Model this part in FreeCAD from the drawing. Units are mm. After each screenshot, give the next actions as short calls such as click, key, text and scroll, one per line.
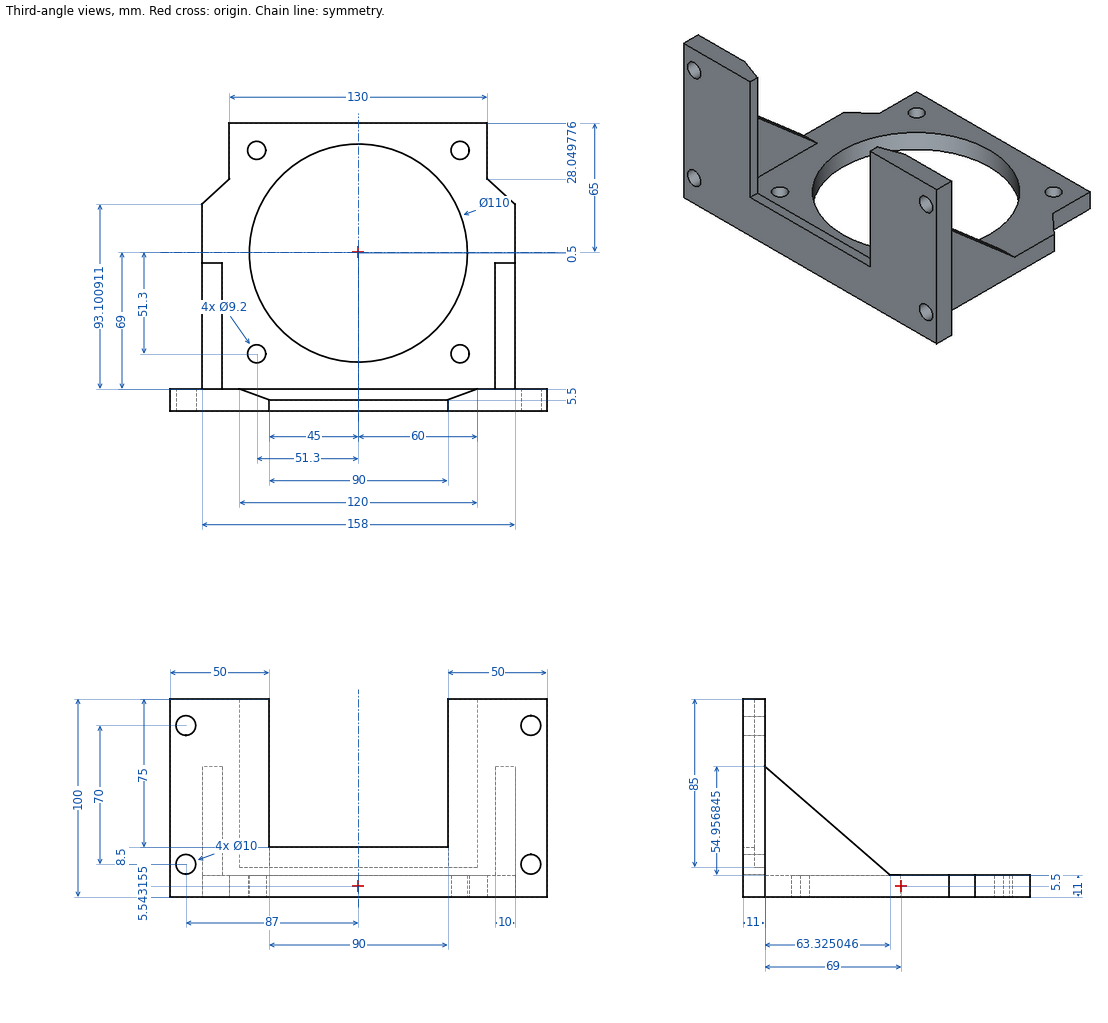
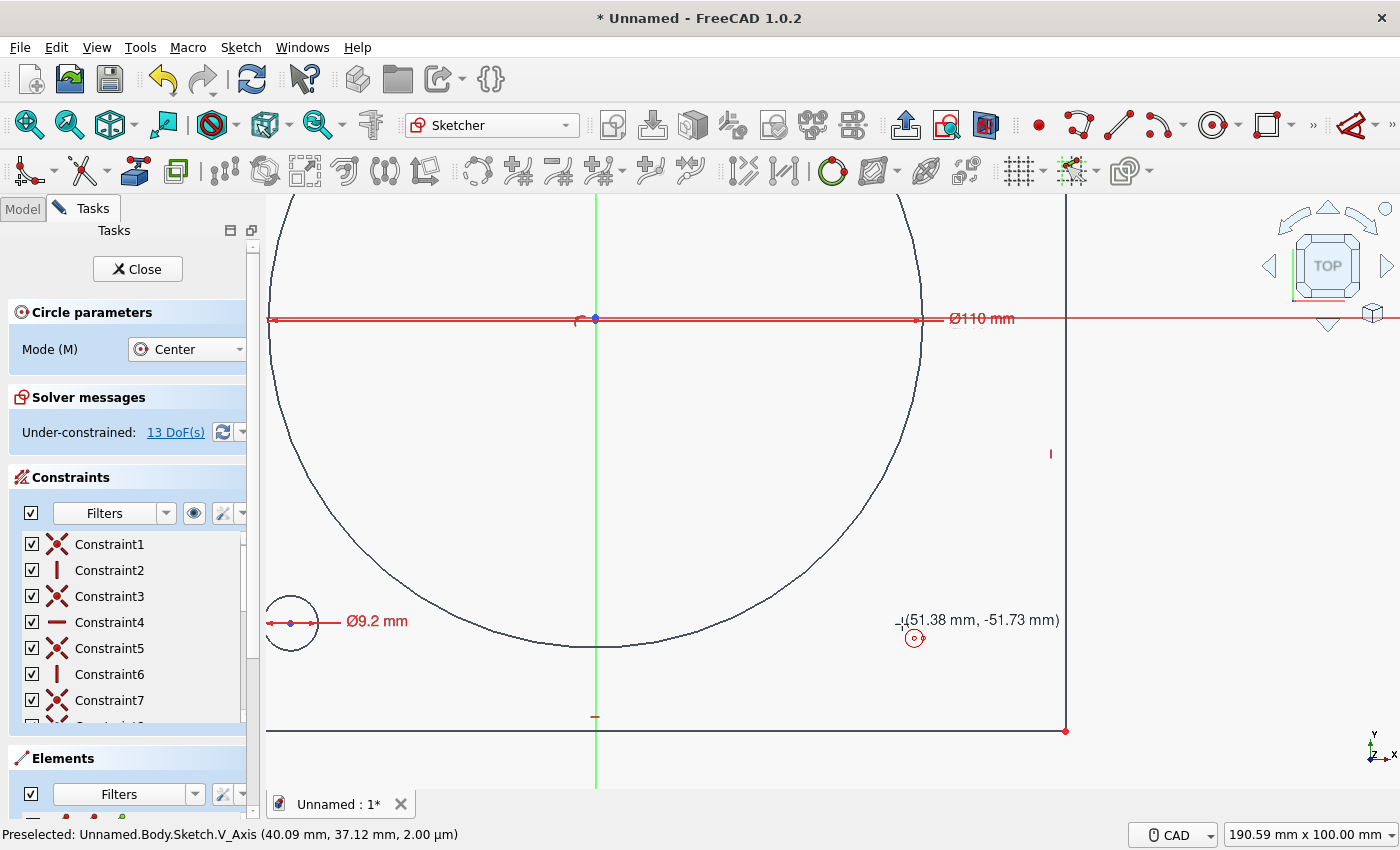
click(901, 623)
move(920, 603)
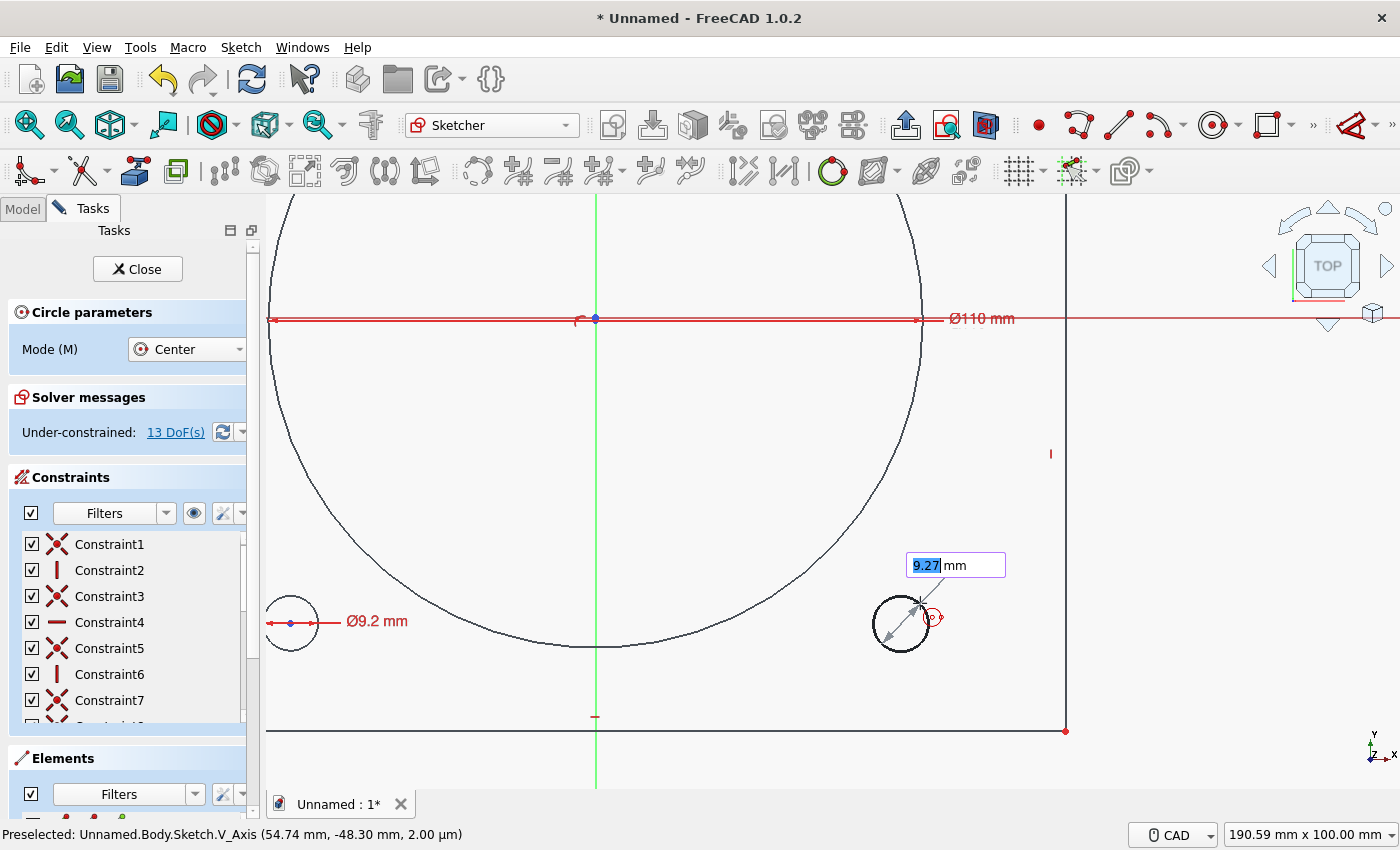
text(9.2)
key(Return)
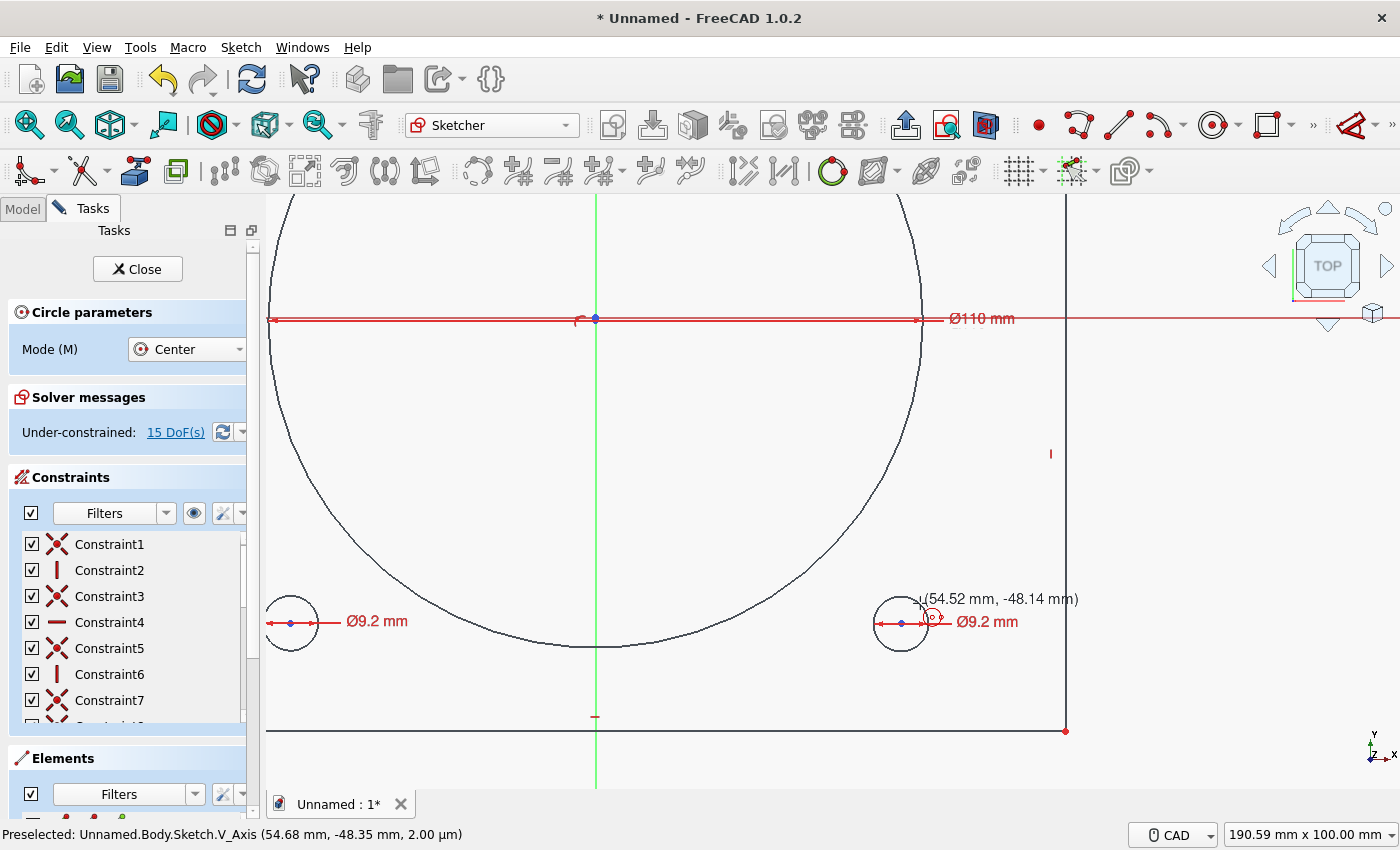
scroll(902, 624, down, 4)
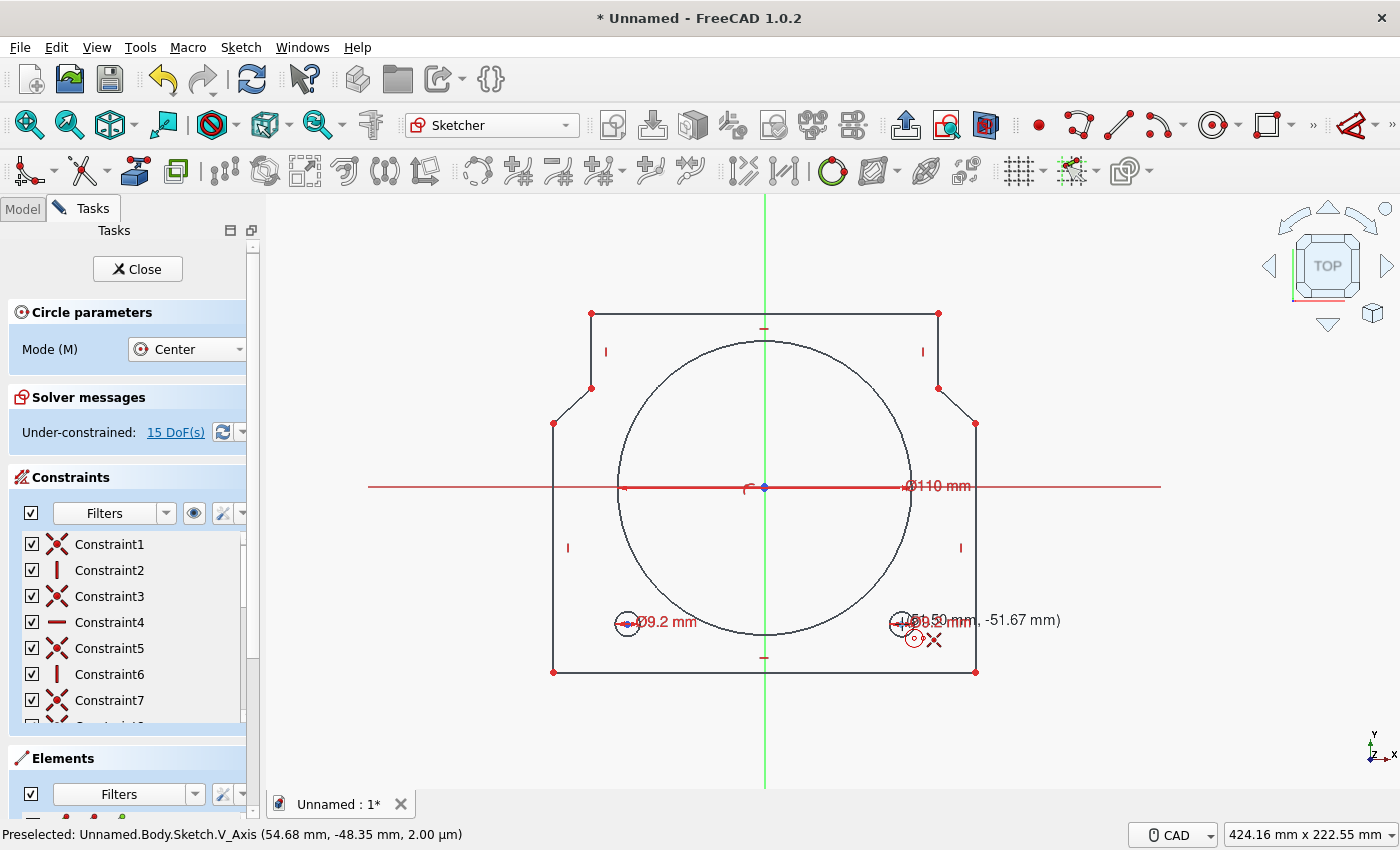
scroll(627, 350, up, 4)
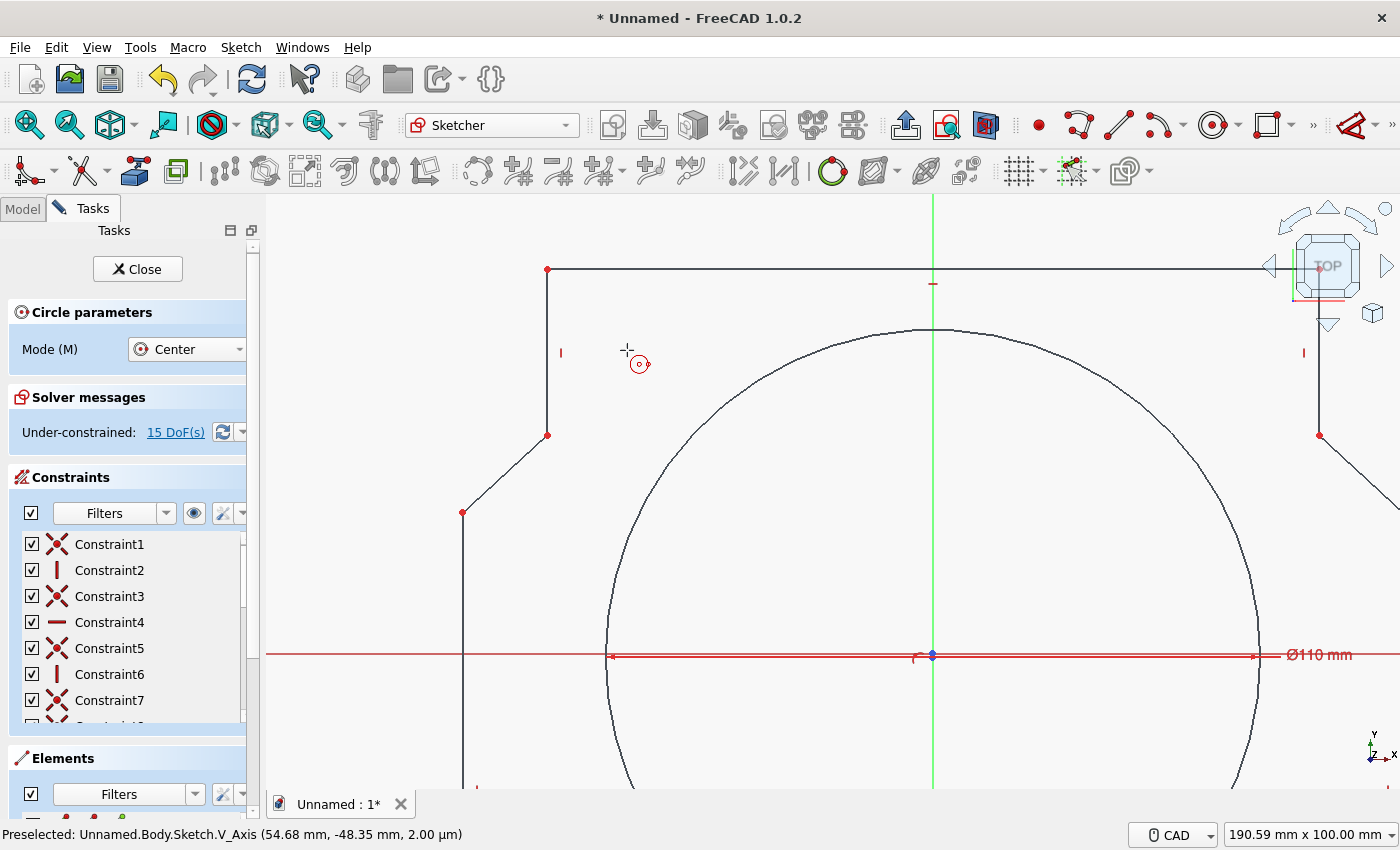
click(628, 349)
move(647, 329)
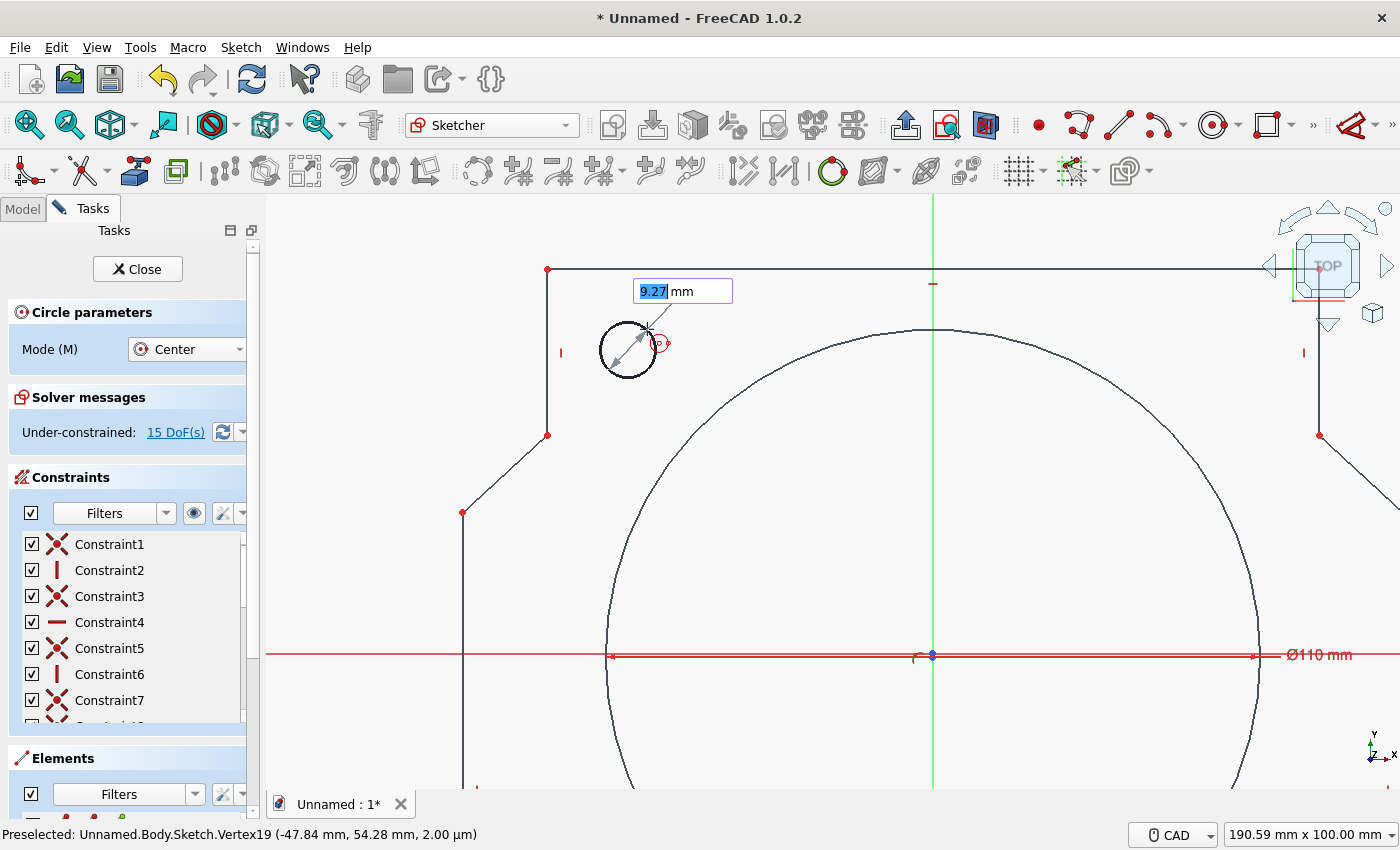
text(9.2)
key(Return)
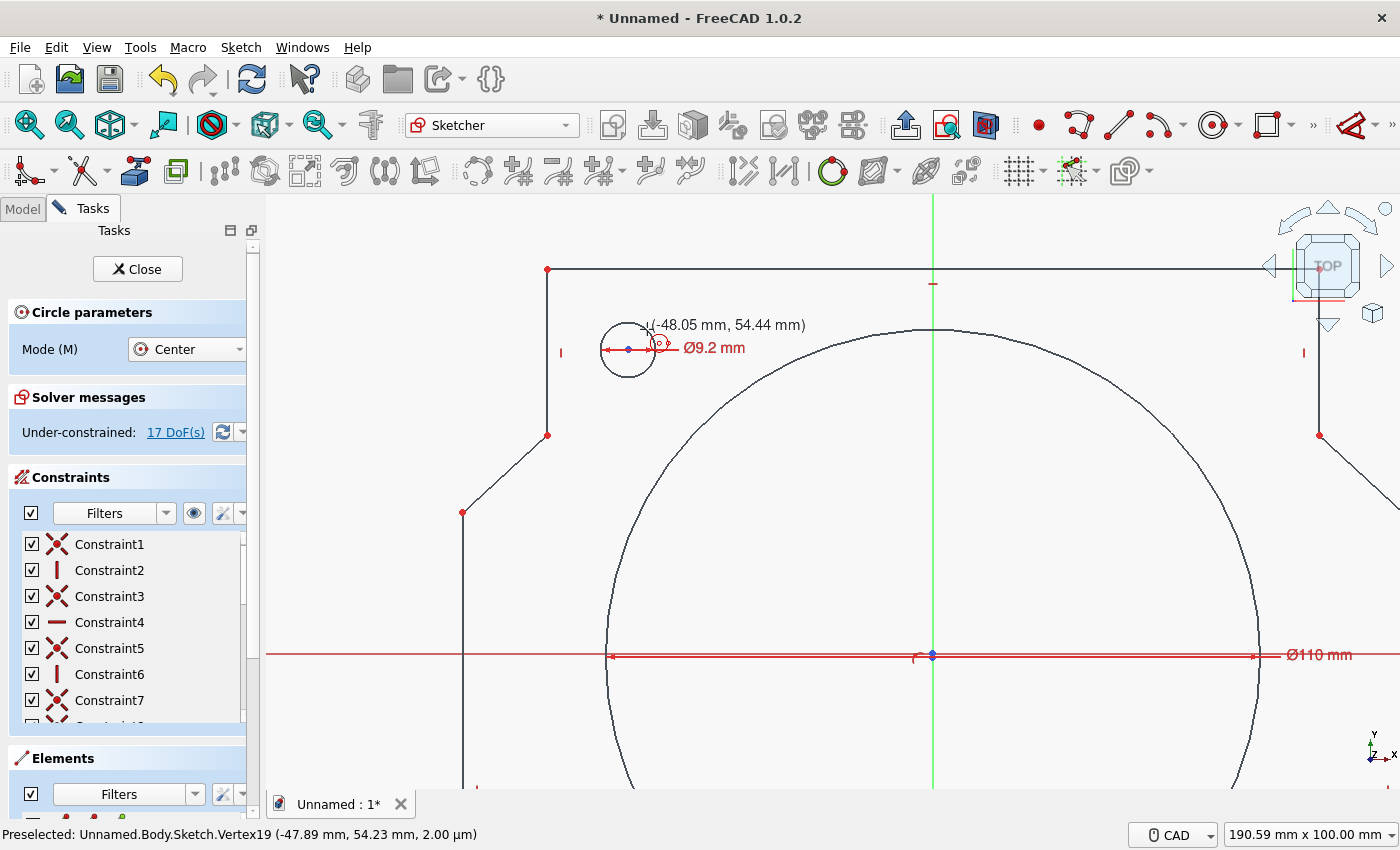
scroll(627, 349, down, 4)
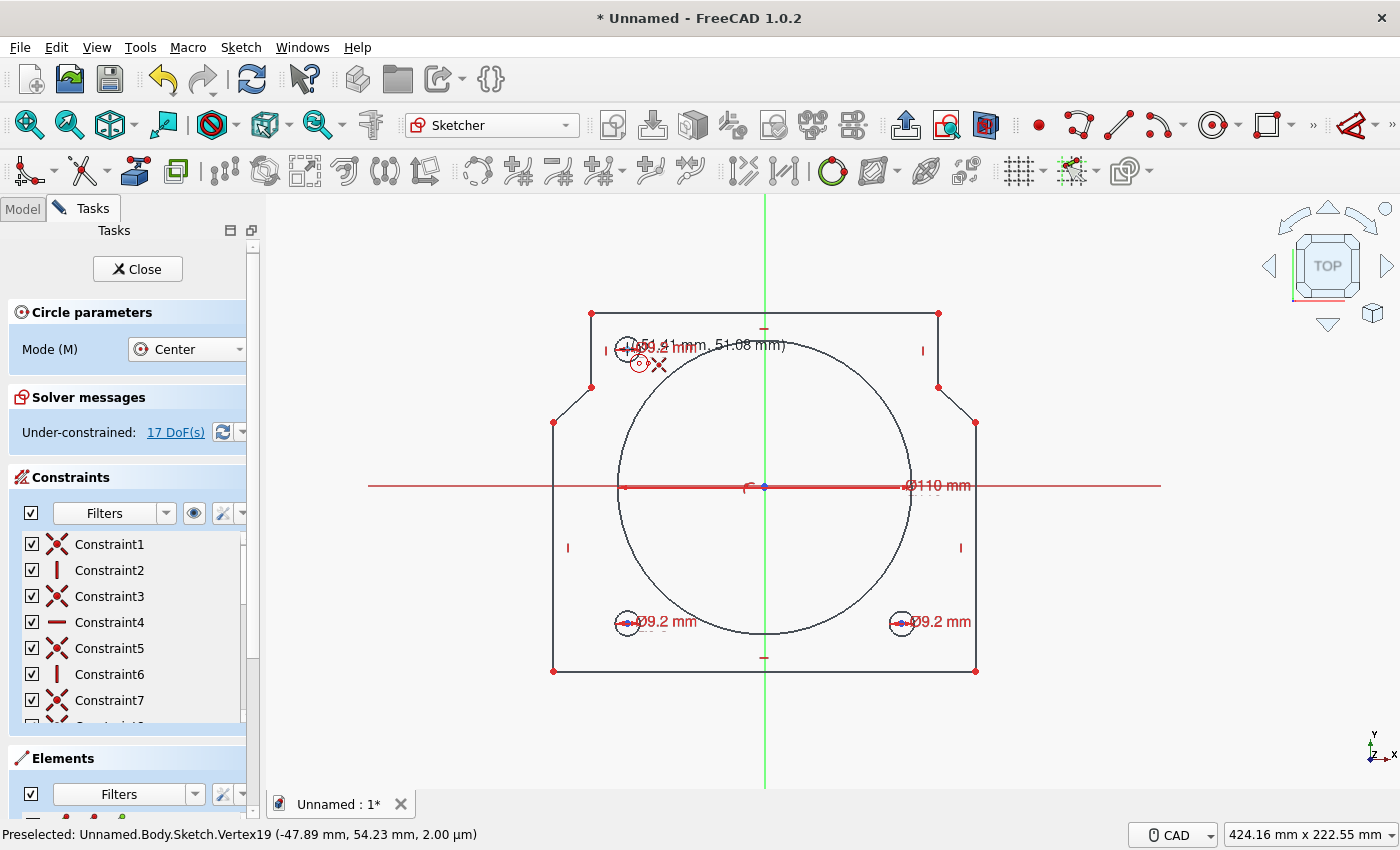
scroll(902, 349, up, 4)